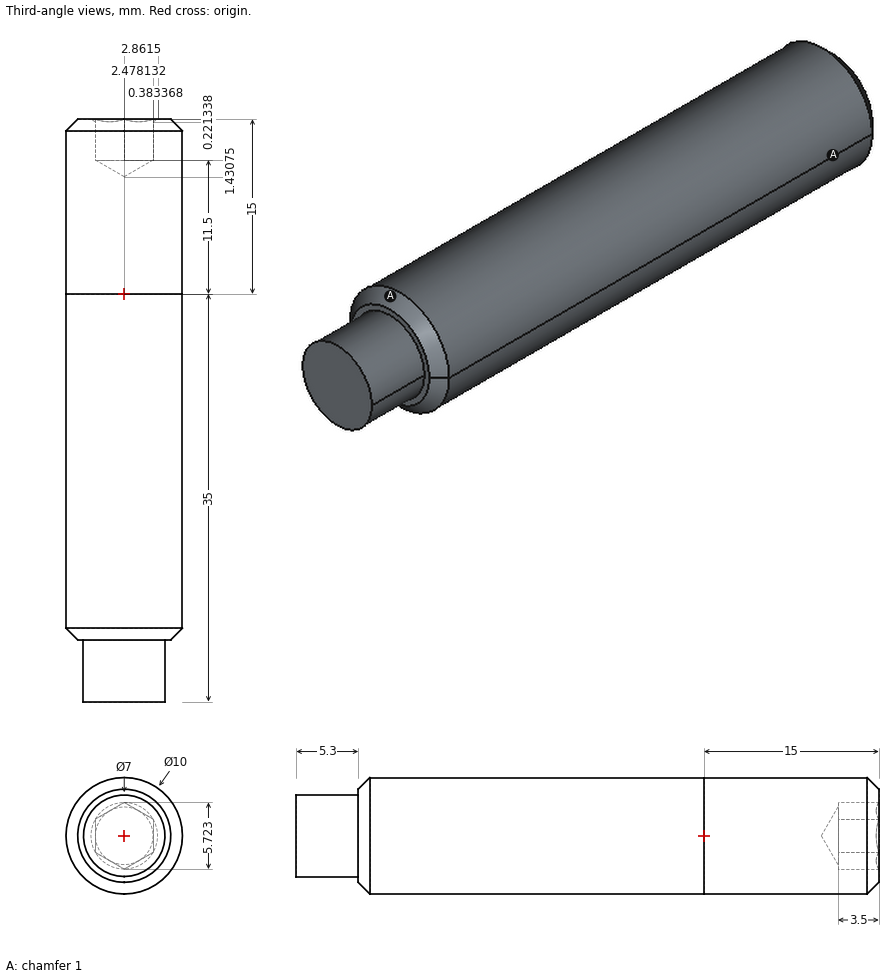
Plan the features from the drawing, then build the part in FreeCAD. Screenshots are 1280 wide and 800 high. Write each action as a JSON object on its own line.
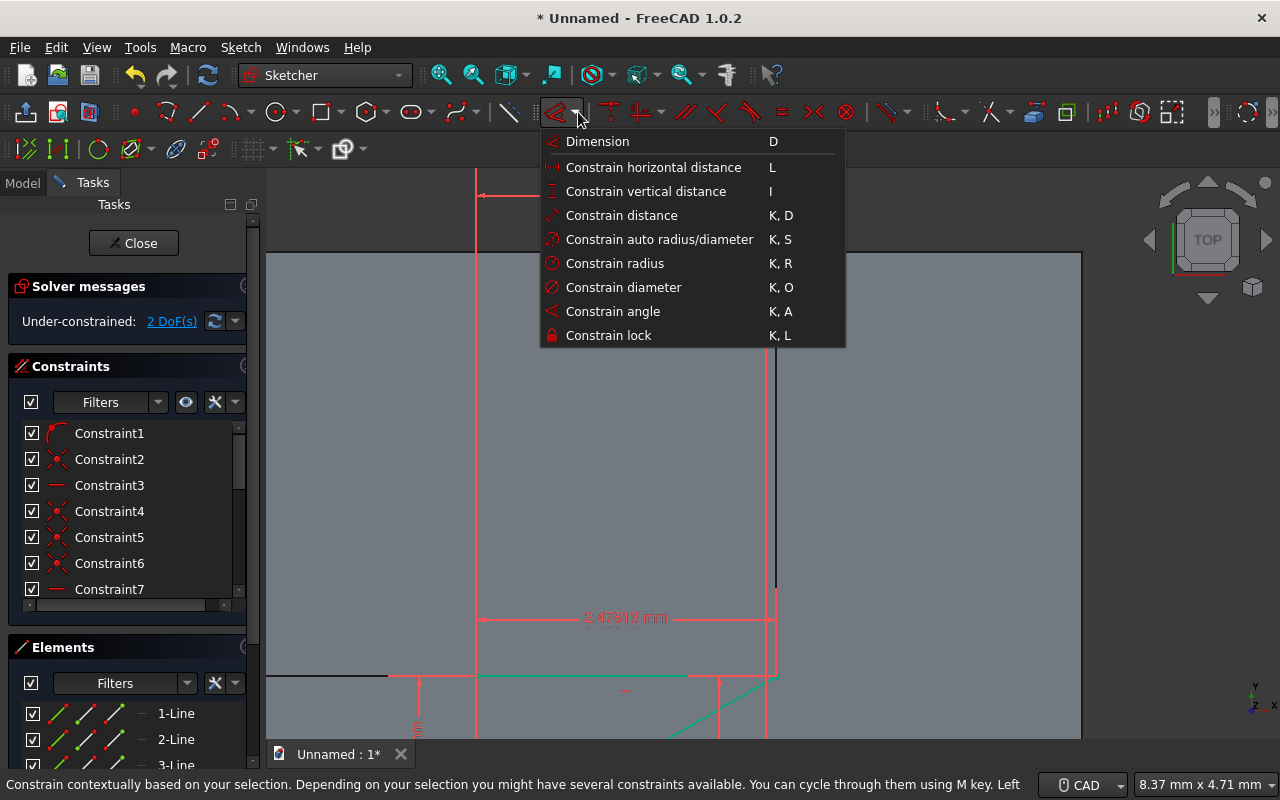
{"action": "left_click", "coordinate": [693, 167]}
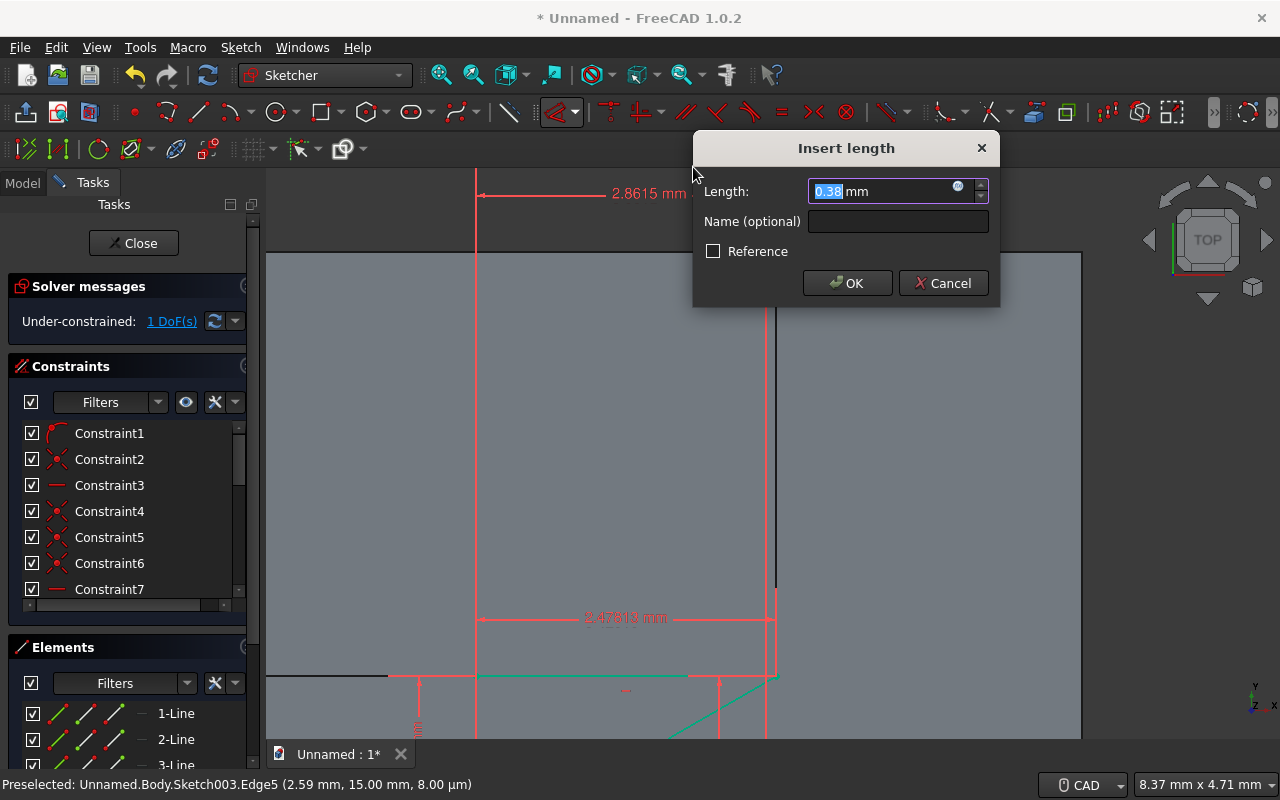
{"action": "type", "text": "0.383368"}
{"action": "key", "text": "Return"}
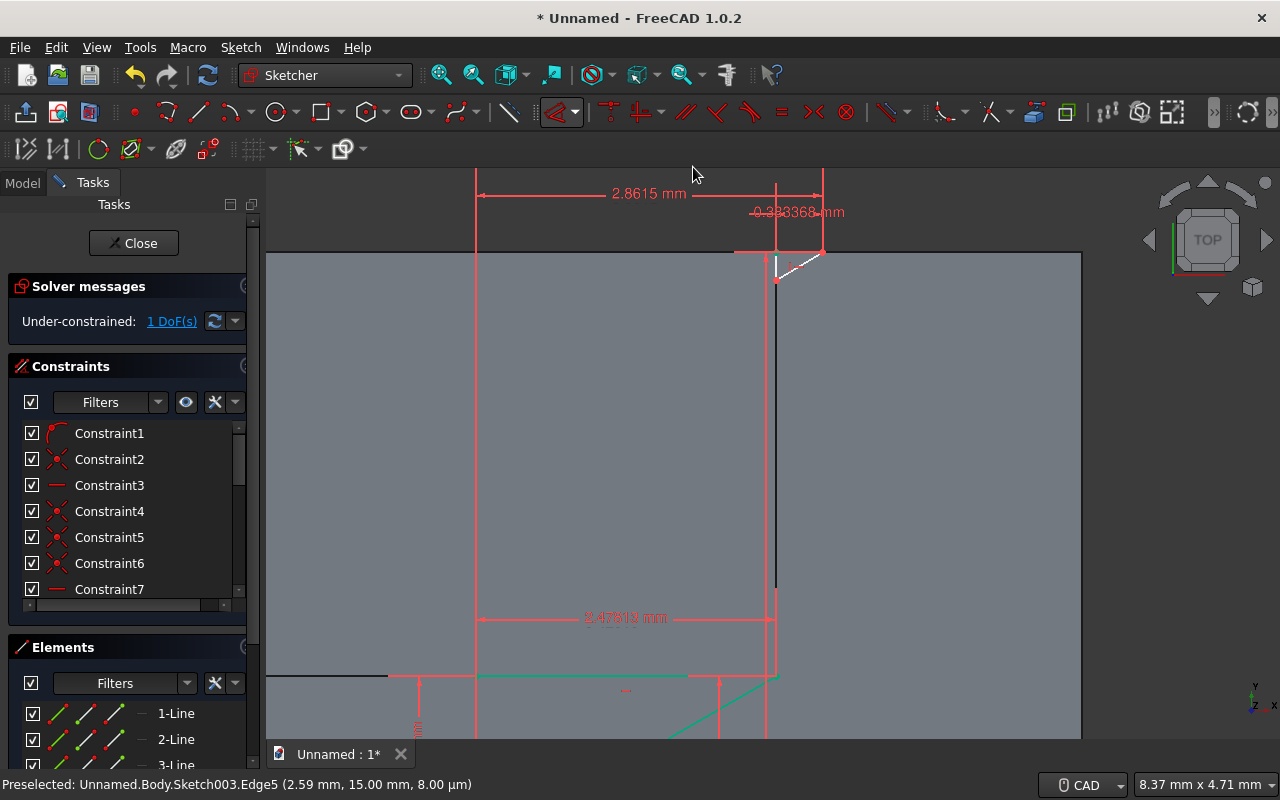
{"action": "scroll", "coordinate": [776, 264], "scroll_direction": "up", "scroll_amount": 2}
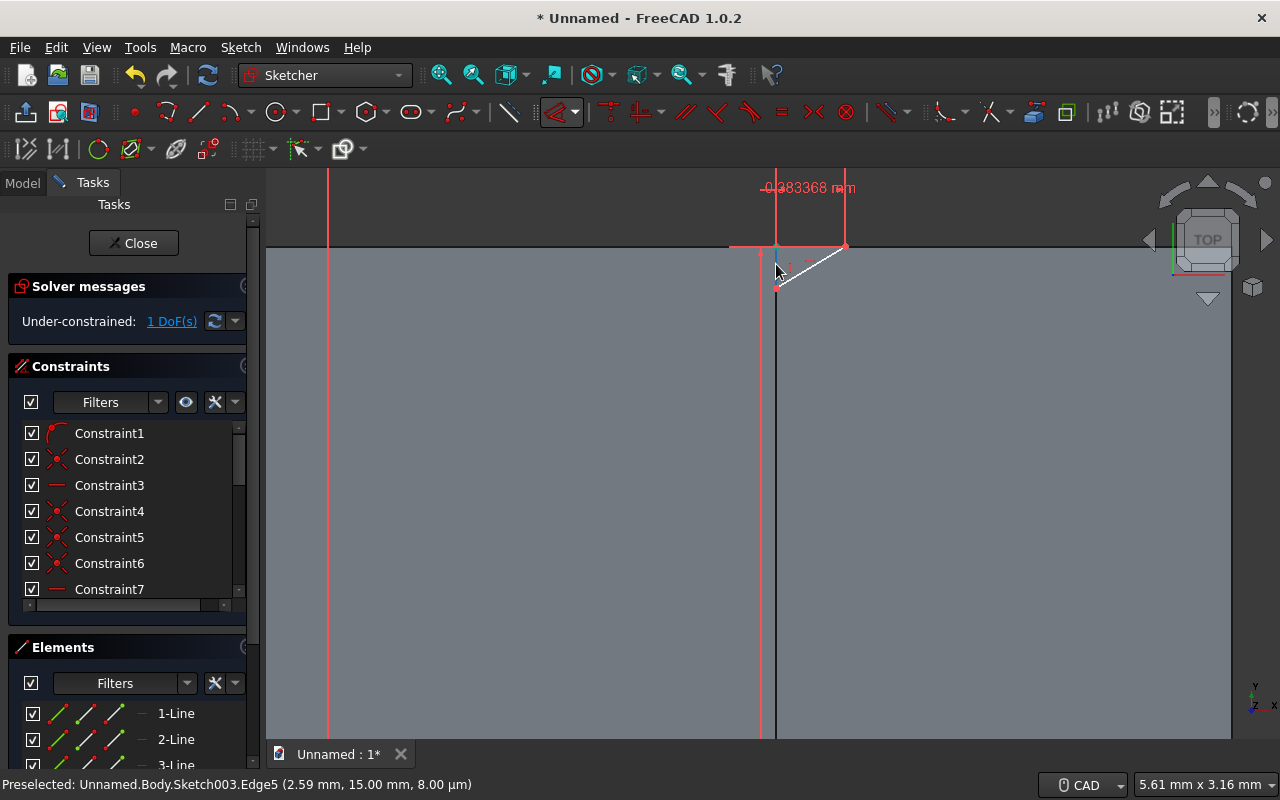
{"action": "left_click", "coordinate": [776, 263]}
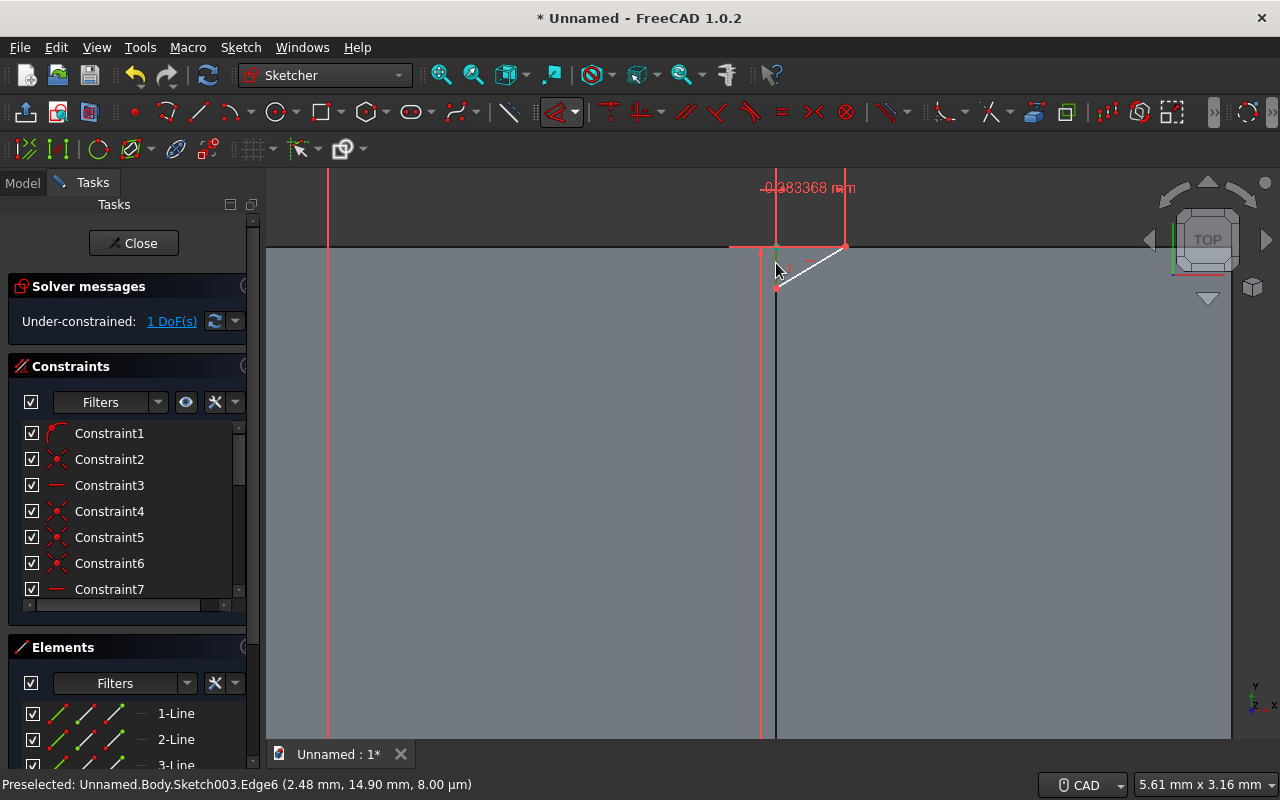
{"action": "left_click", "coordinate": [578, 112]}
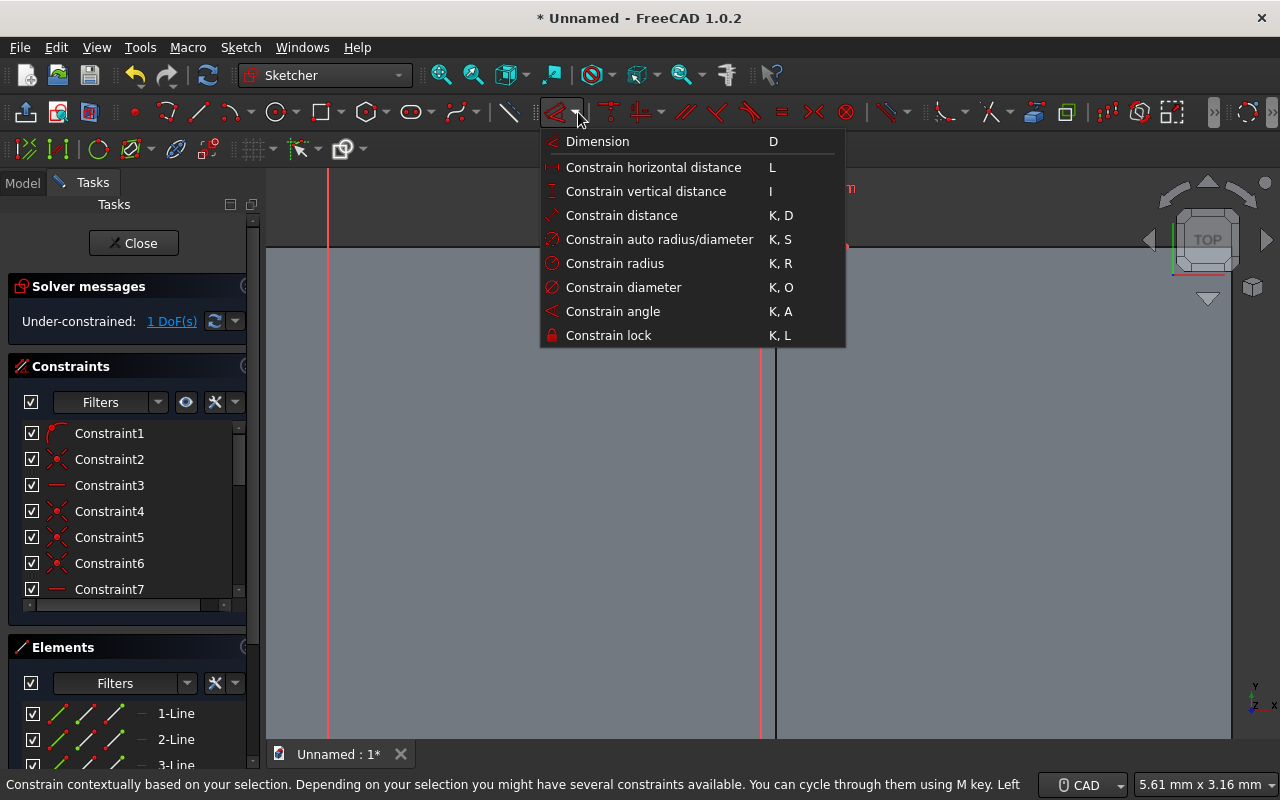
{"action": "left_click", "coordinate": [693, 191]}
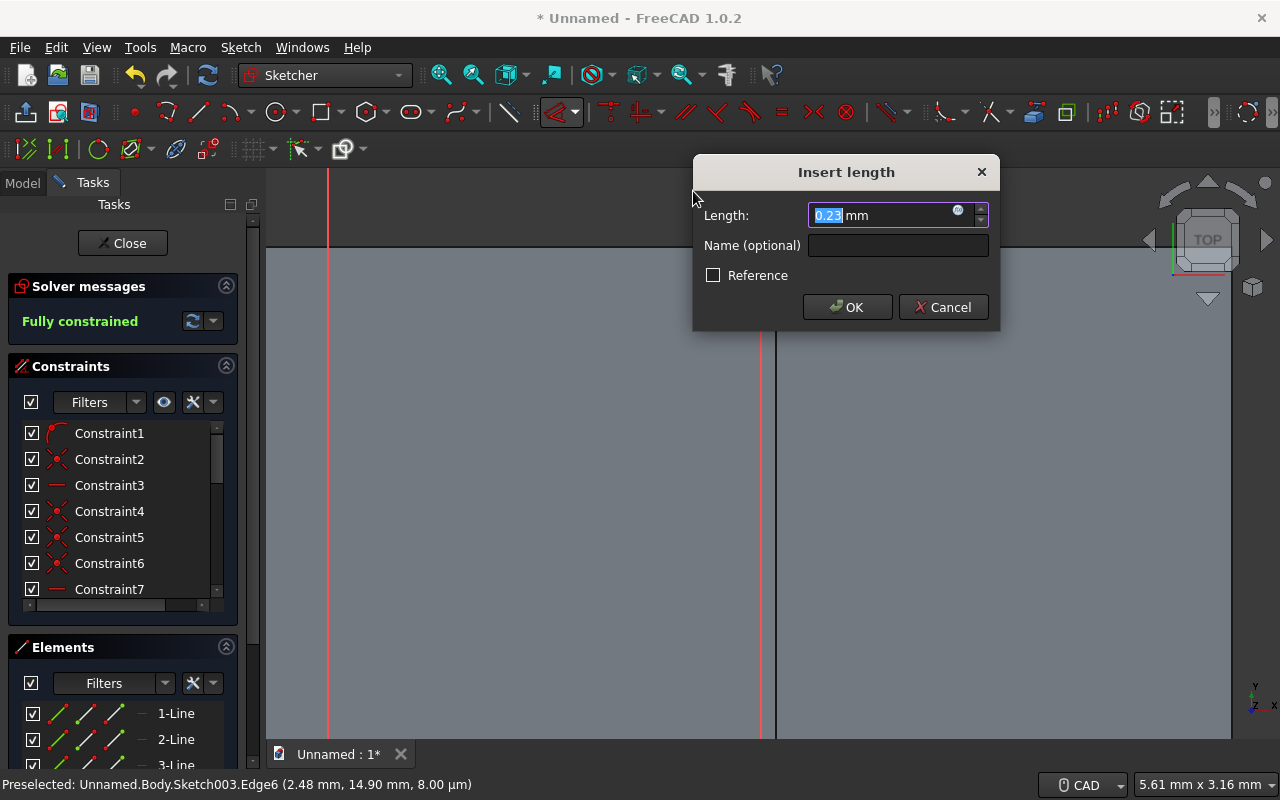
{"action": "type", "text": "0.221338"}
{"action": "key", "text": "Return"}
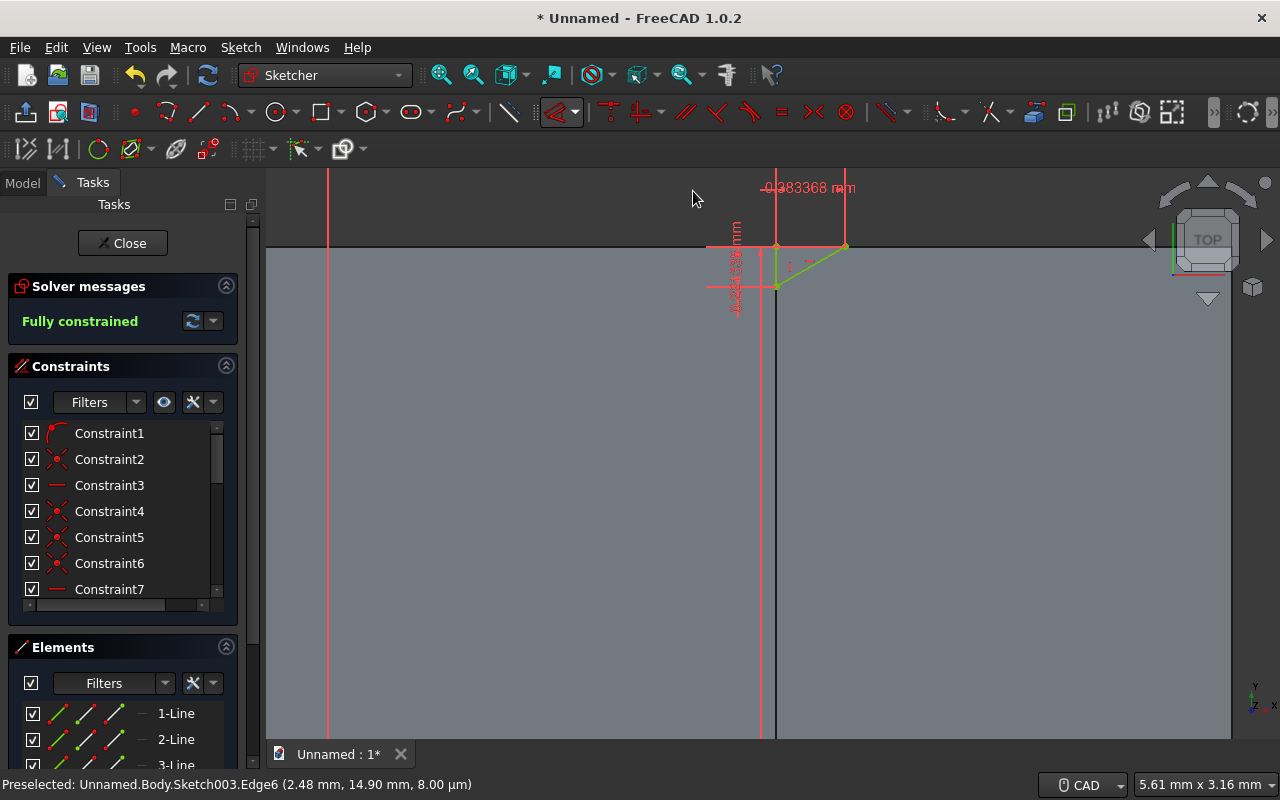
{"action": "left_click", "coordinate": [123, 243]}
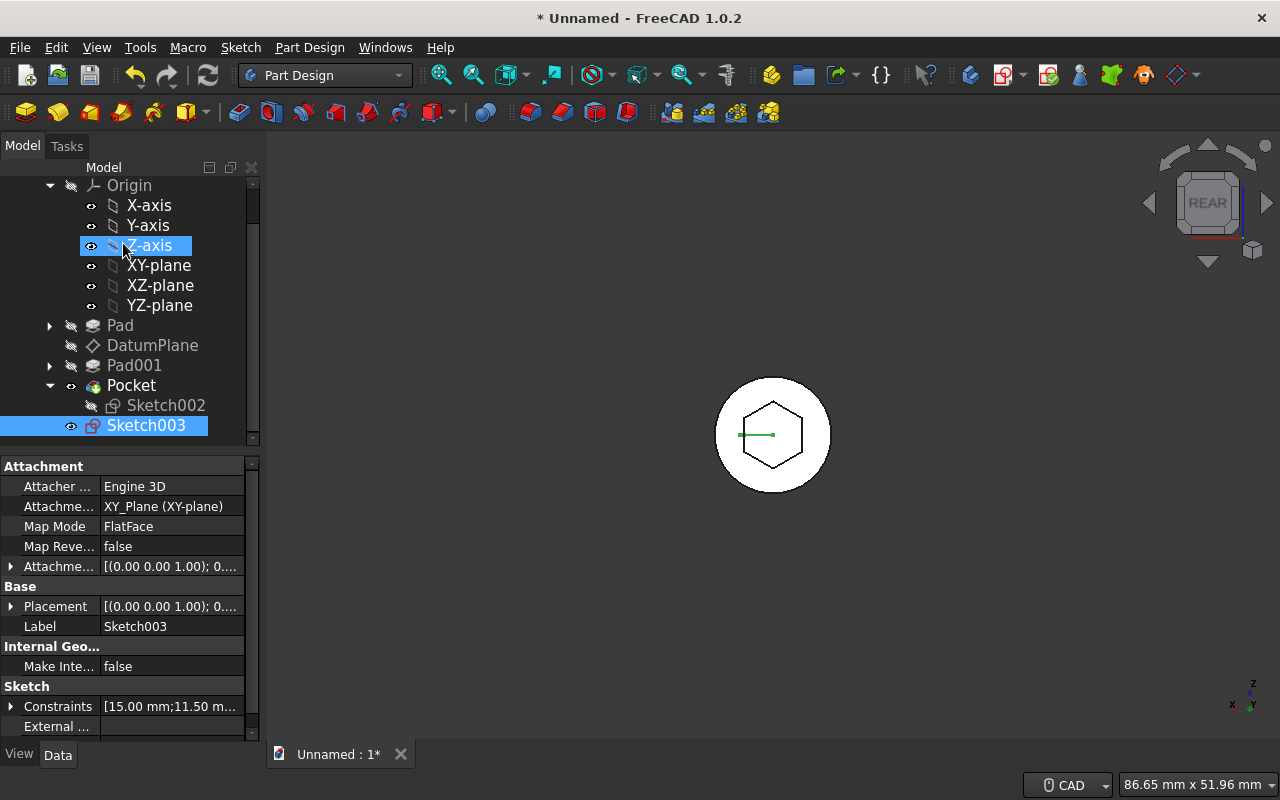
{"action": "left_click", "coordinate": [304, 112]}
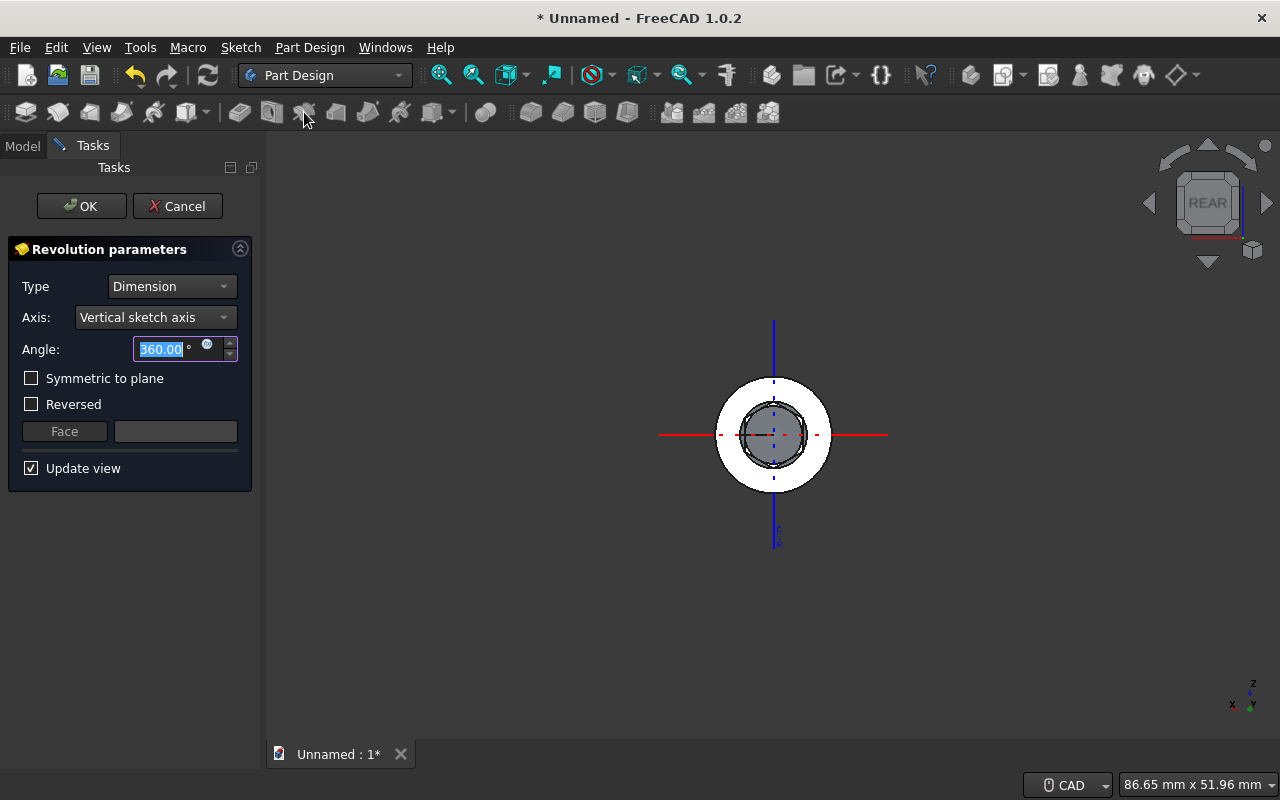
{"action": "left_click", "coordinate": [82, 206]}